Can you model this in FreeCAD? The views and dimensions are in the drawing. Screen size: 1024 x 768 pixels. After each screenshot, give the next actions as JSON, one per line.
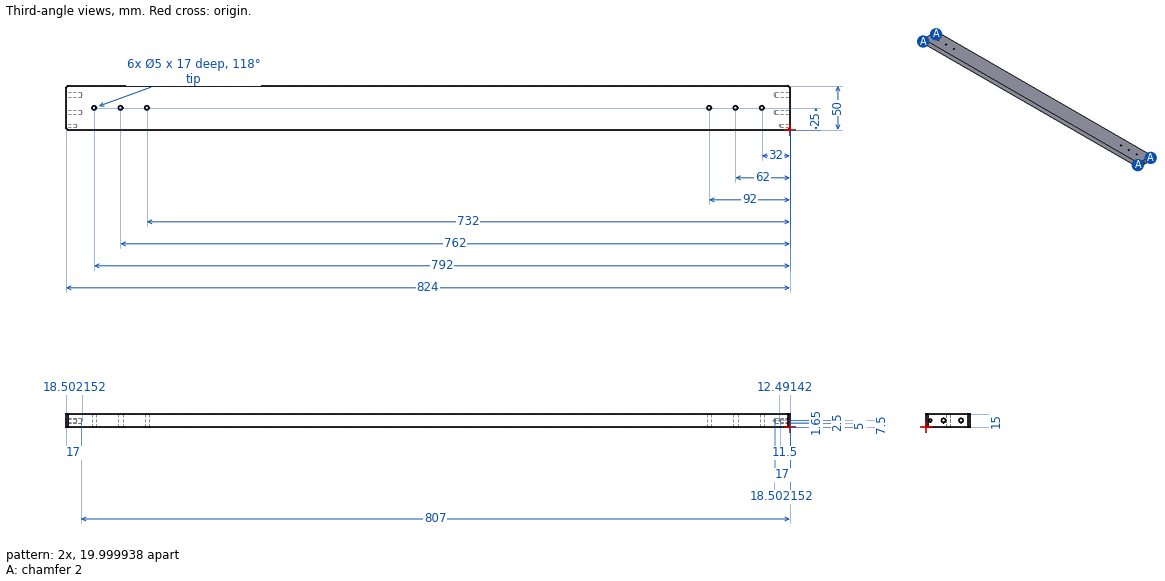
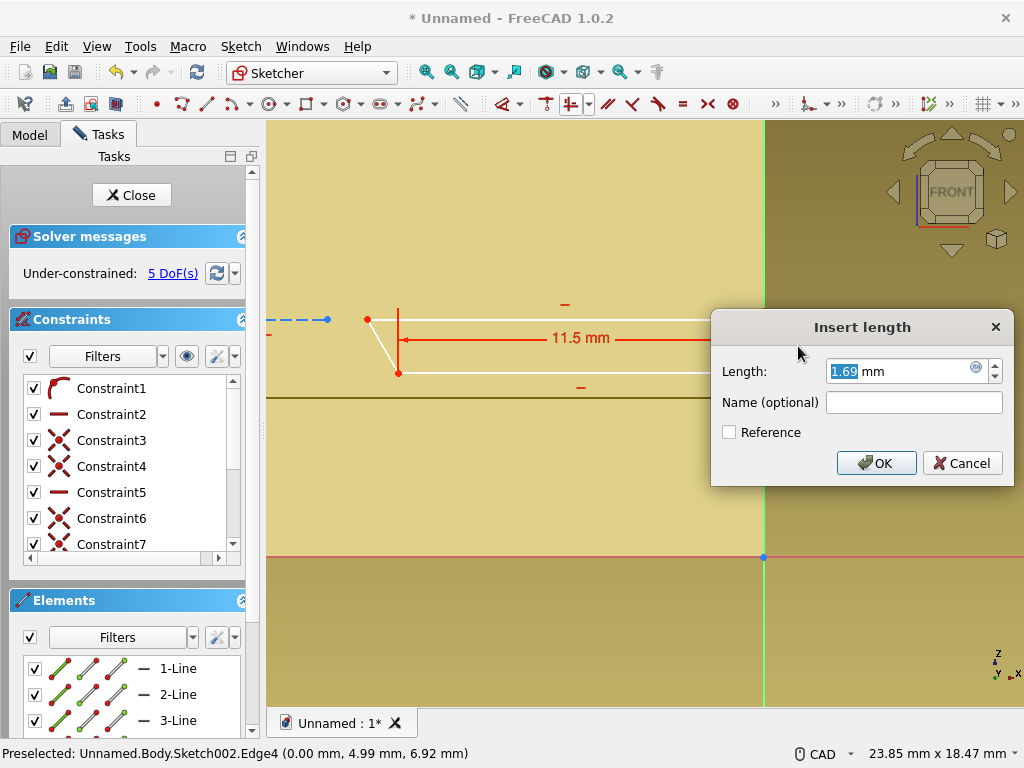
{"action": "type", "text": "1.65"}
{"action": "key", "text": "Return"}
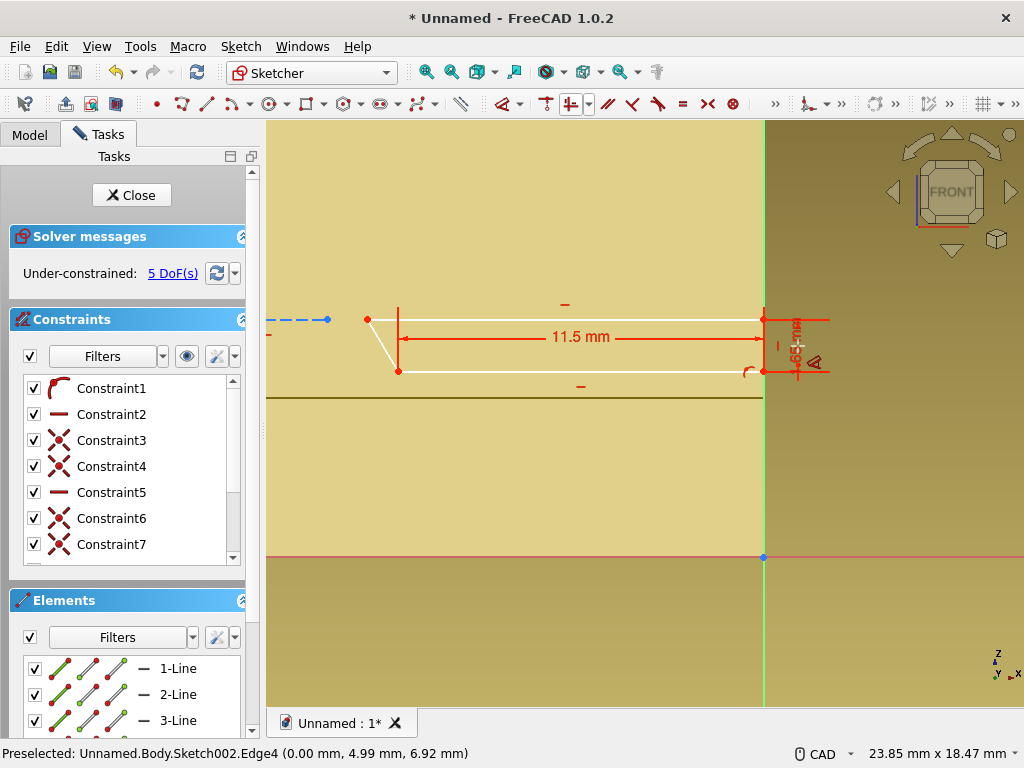
{"action": "left_click", "coordinate": [367, 320]}
{"action": "left_click", "coordinate": [798, 438]}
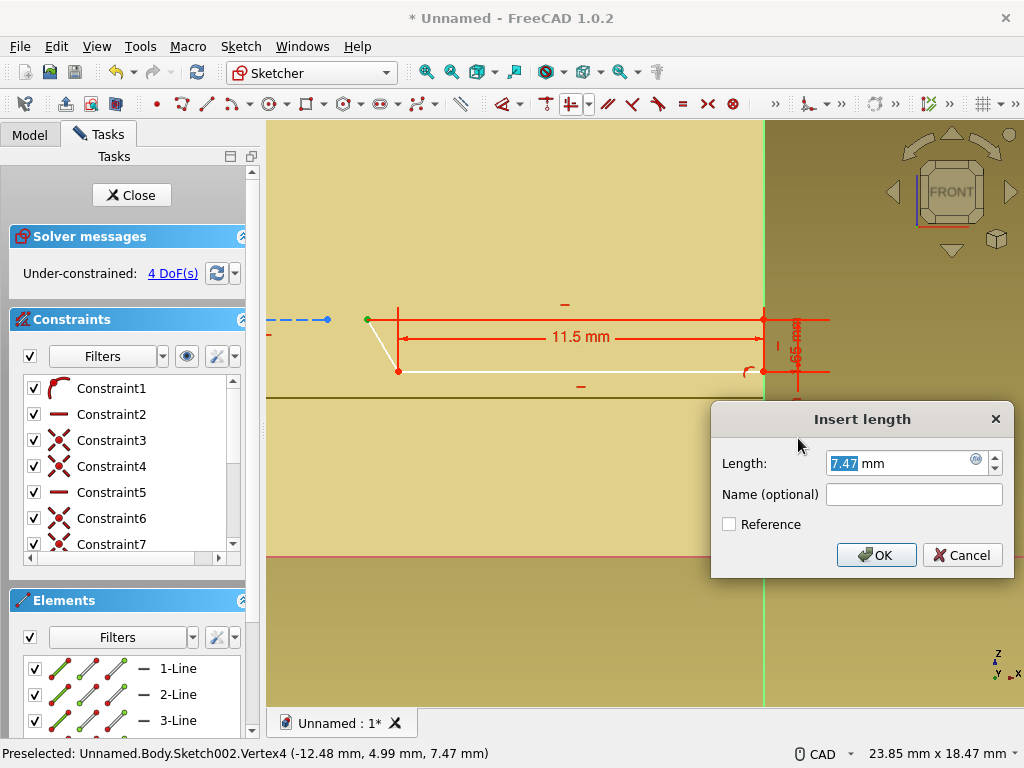
{"action": "type", "text": "7.5"}
{"action": "key", "text": "Return"}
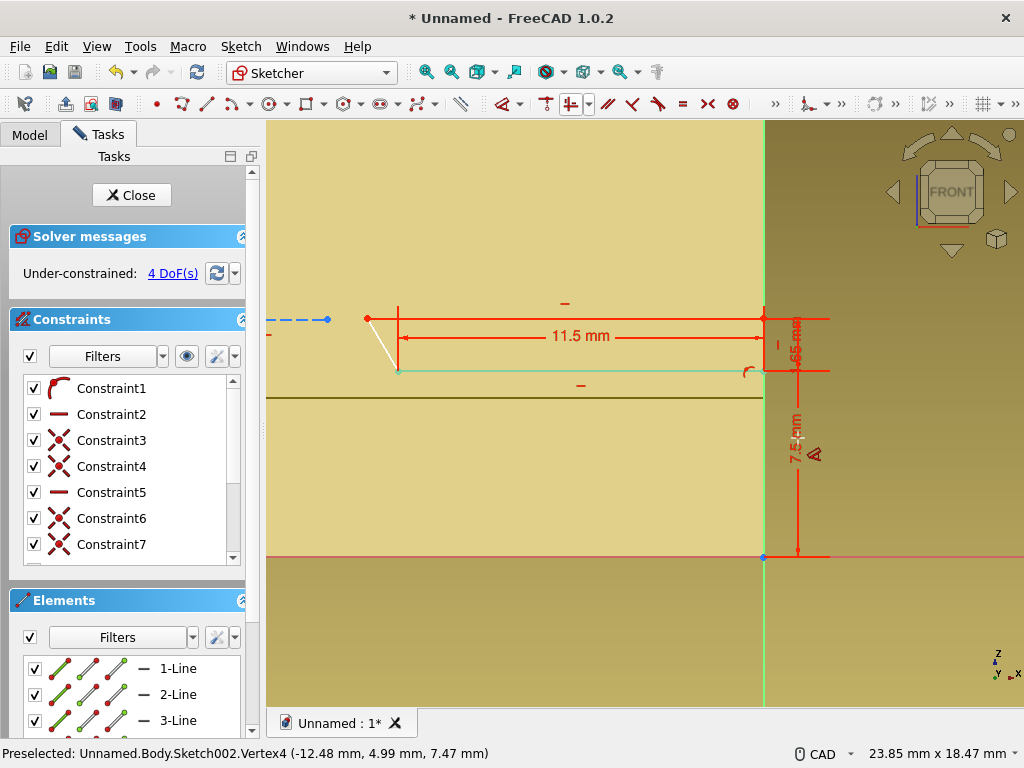
{"action": "left_click", "coordinate": [327, 320]}
{"action": "left_click", "coordinate": [798, 384]}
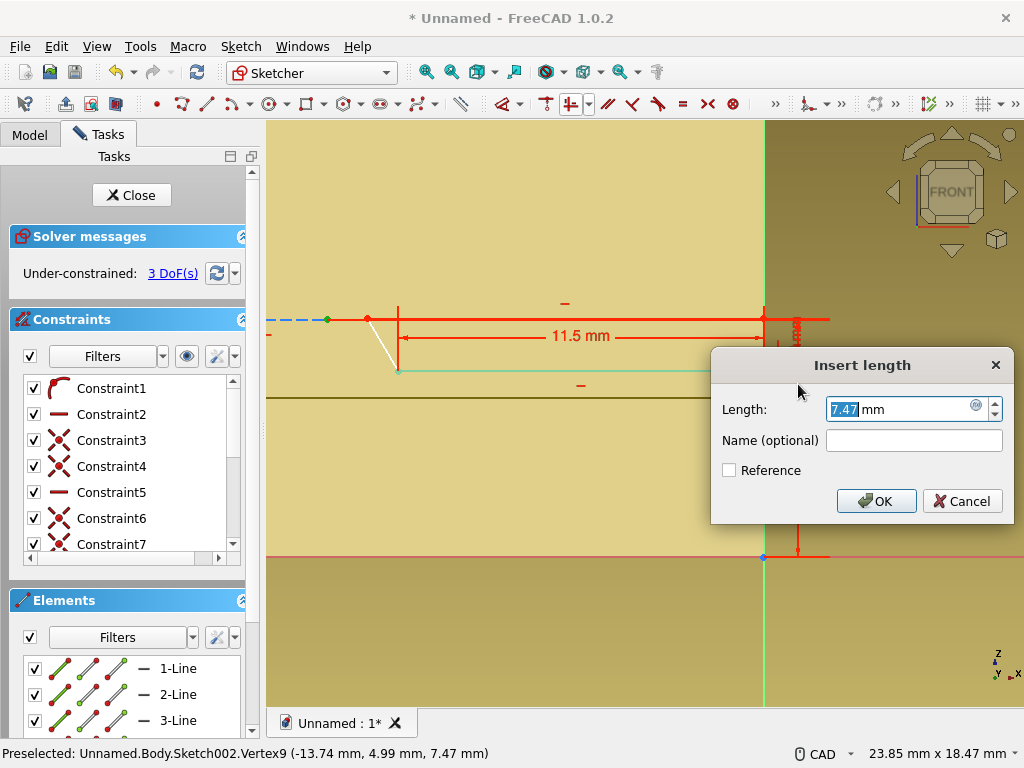
{"action": "type", "text": "7.5"}
{"action": "key", "text": "Return"}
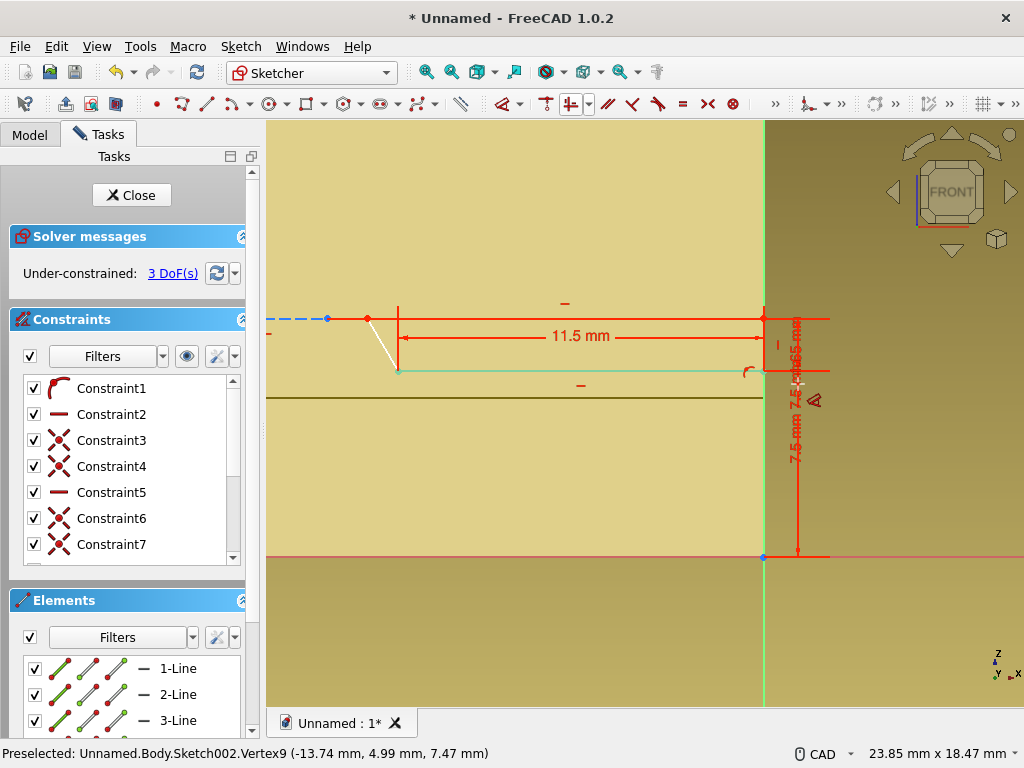
{"action": "left_click", "coordinate": [486, 319]}
{"action": "left_click", "coordinate": [566, 285]}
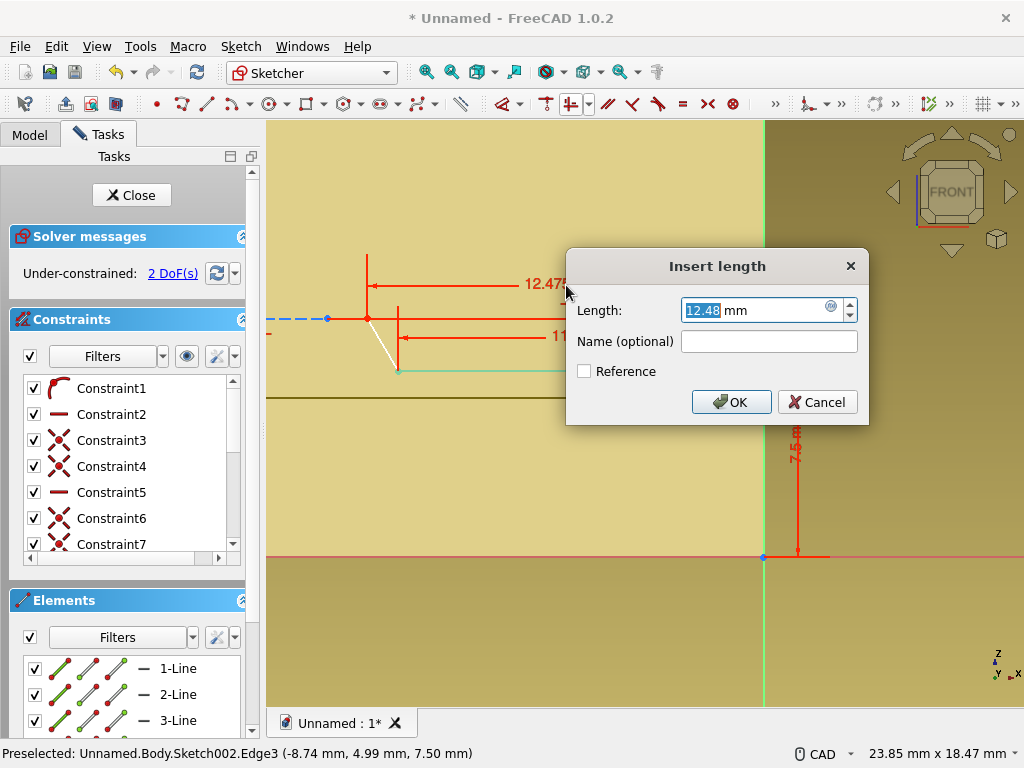
{"action": "type", "text": "12.49142"}
{"action": "key", "text": "Return"}
{"action": "key", "text": "Escape"}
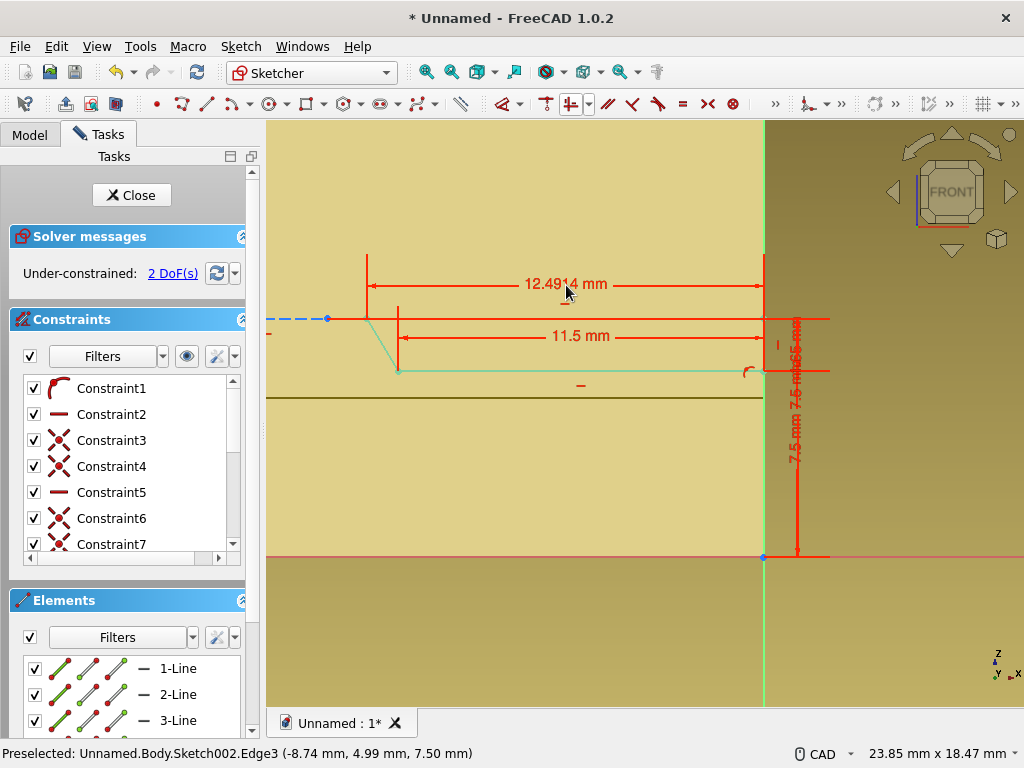
{"action": "left_click", "coordinate": [132, 195]}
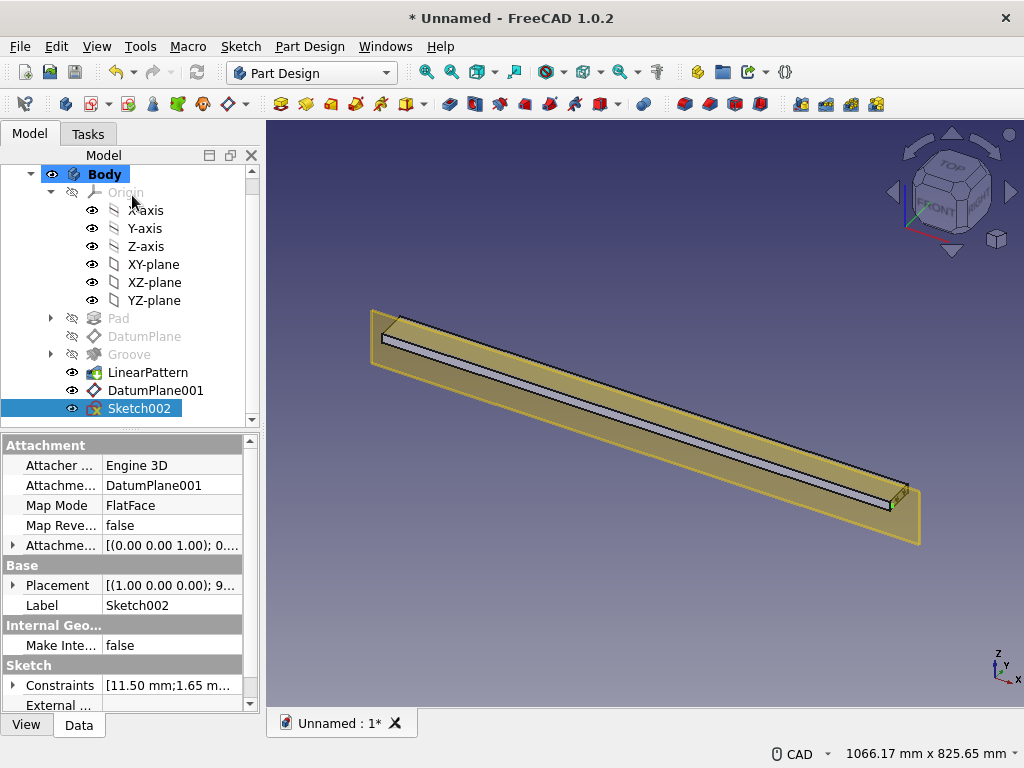
{"action": "left_click", "coordinate": [500, 104]}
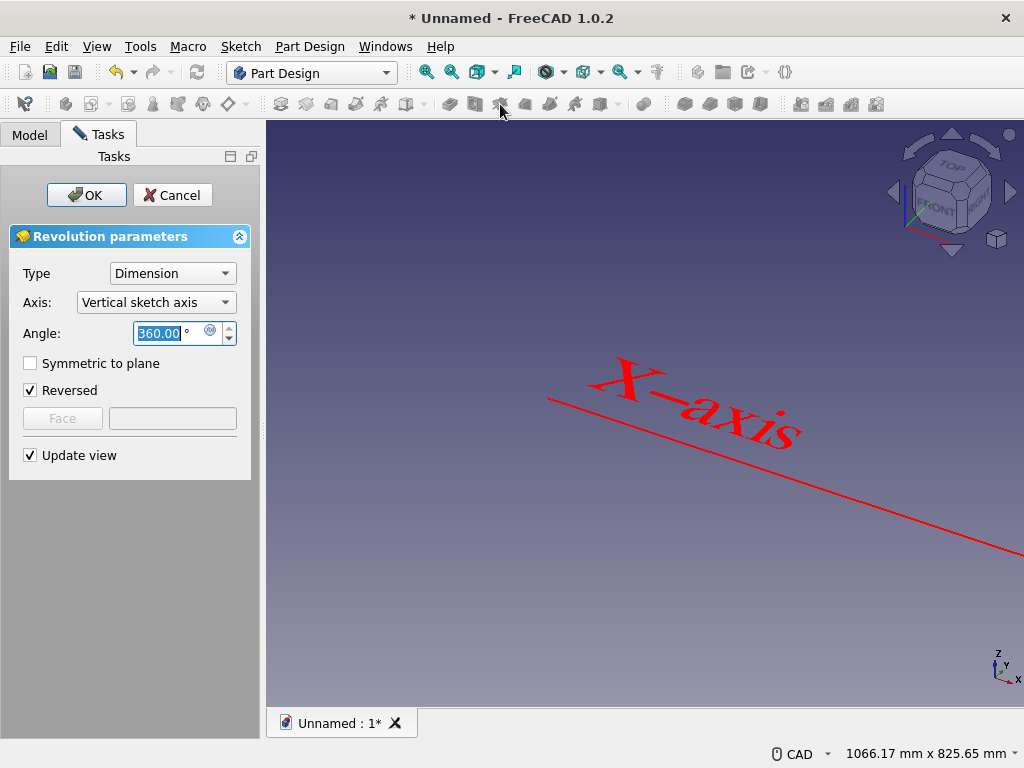
{"action": "left_click", "coordinate": [157, 302]}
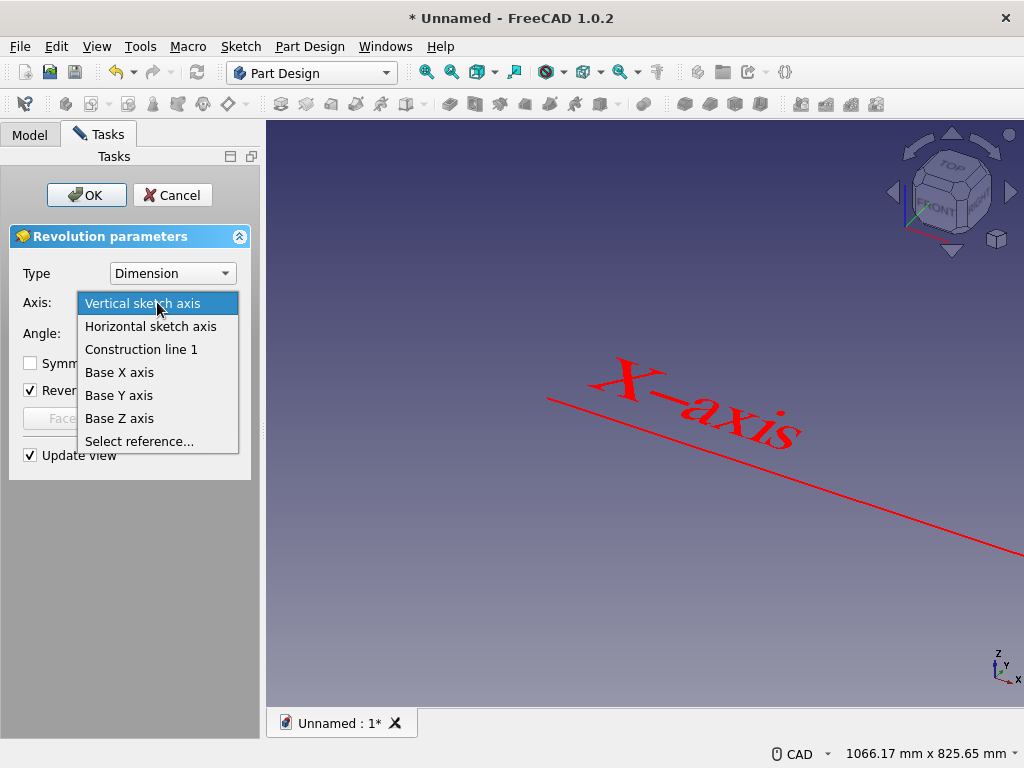
{"action": "left_click", "coordinate": [156, 350]}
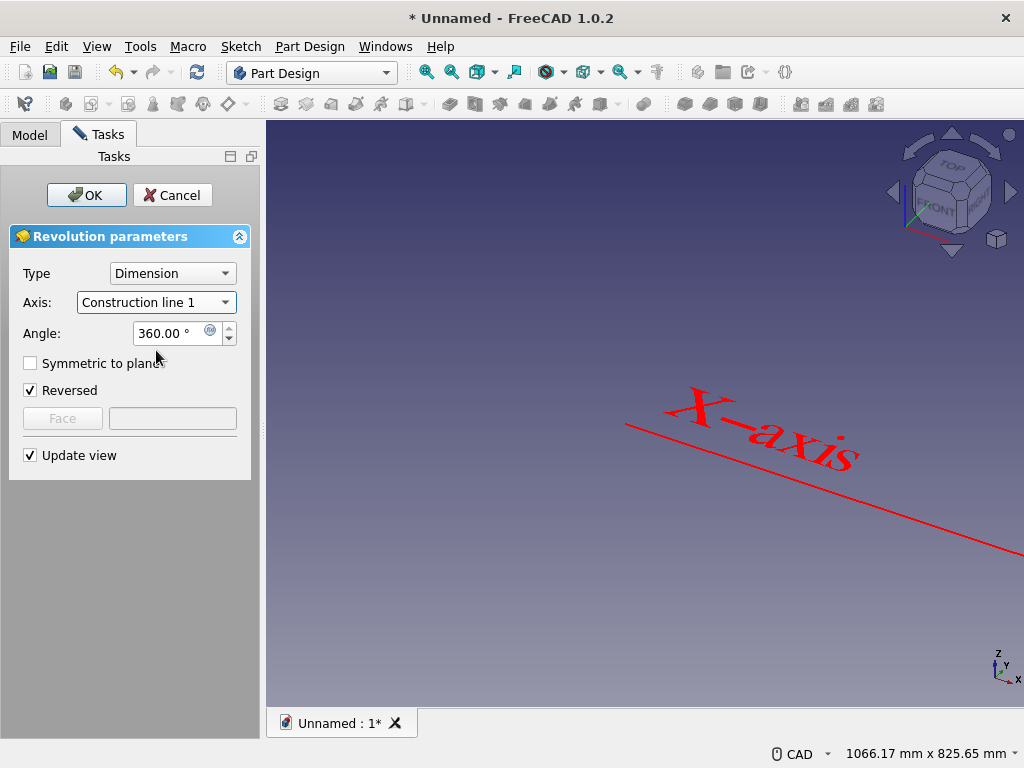
{"action": "left_click", "coordinate": [87, 195]}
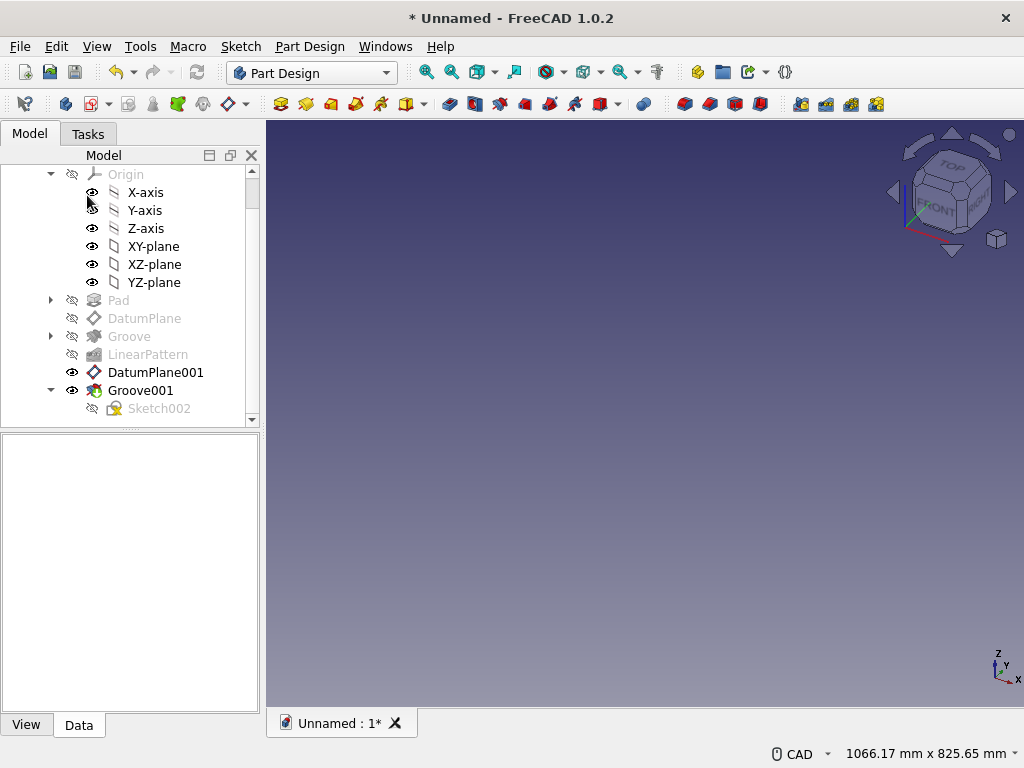
{"action": "left_click", "coordinate": [117, 372]}
{"action": "key", "text": "space"}